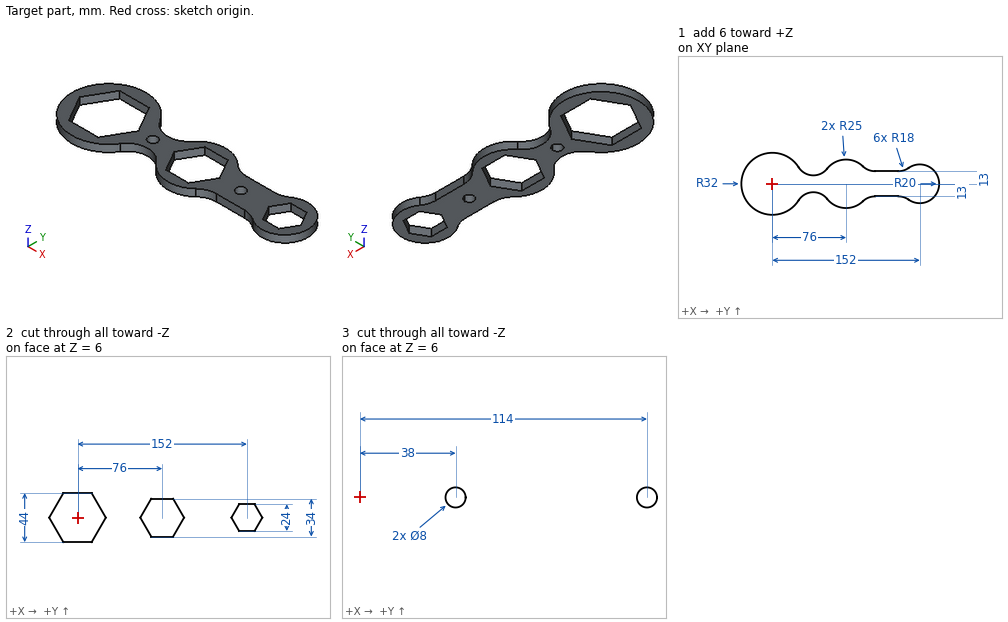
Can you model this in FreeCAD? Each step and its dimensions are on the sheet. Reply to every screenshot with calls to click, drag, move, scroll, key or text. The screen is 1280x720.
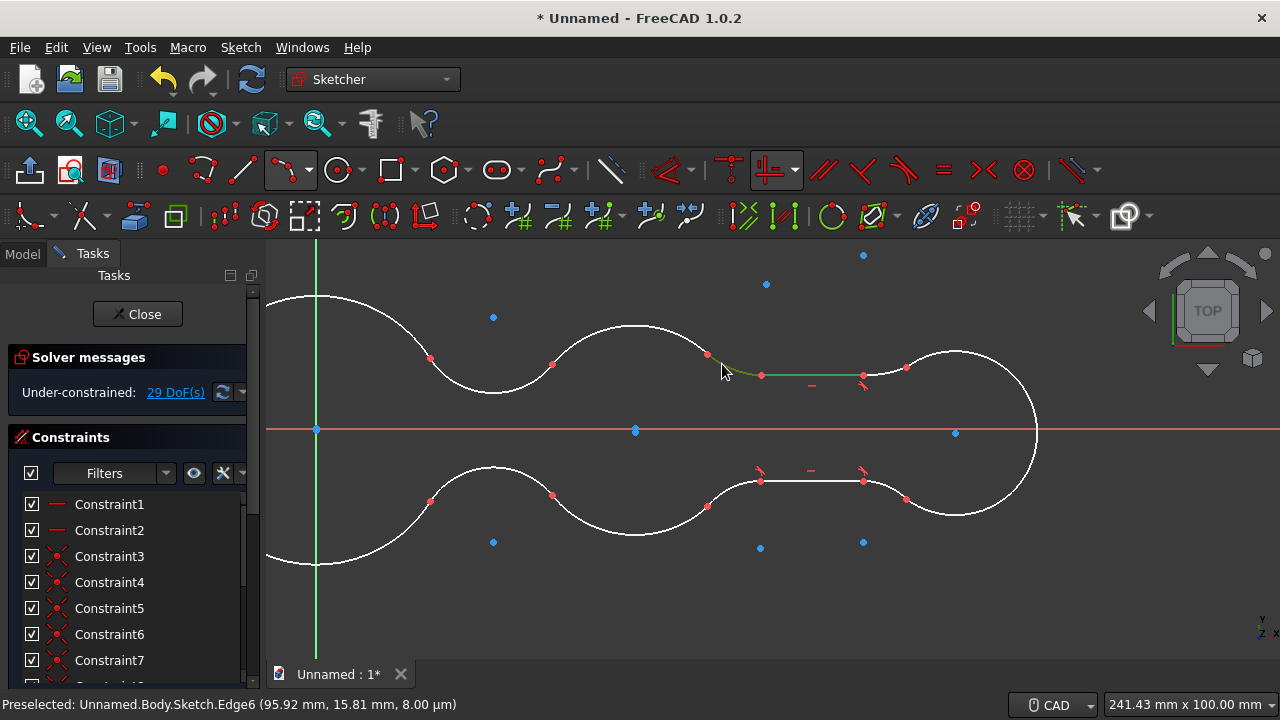
click(904, 170)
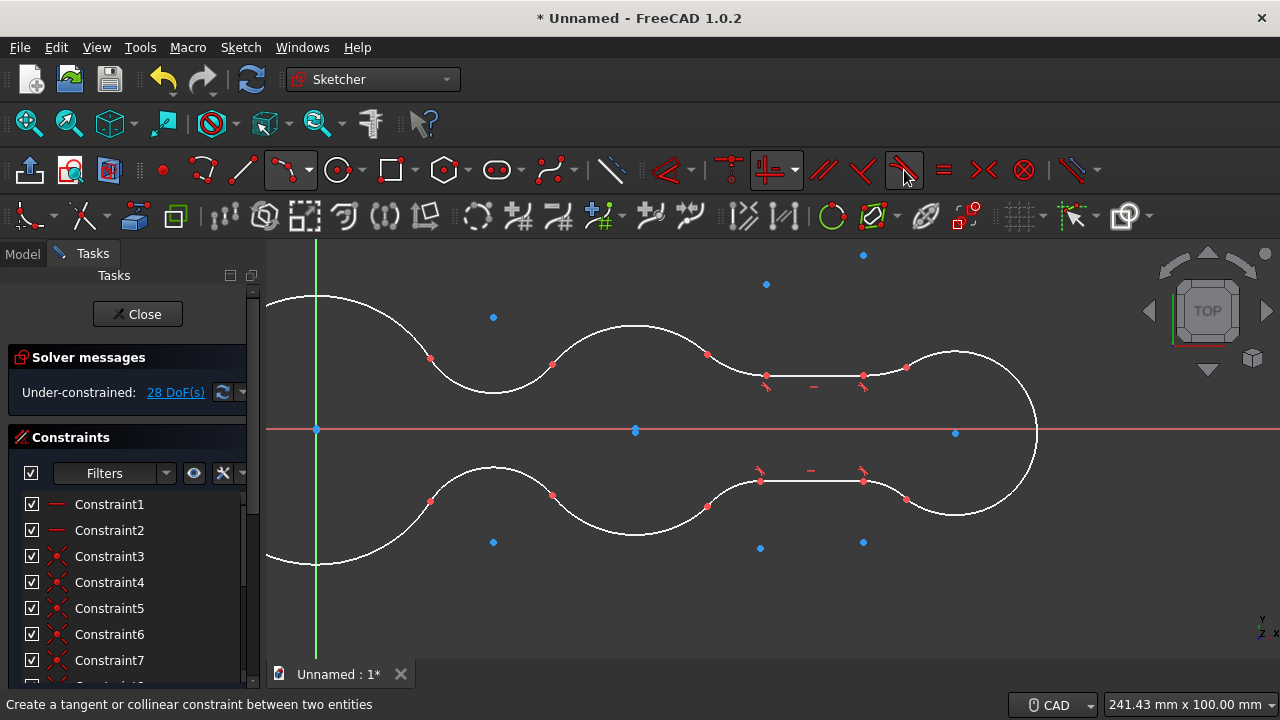
click(895, 490)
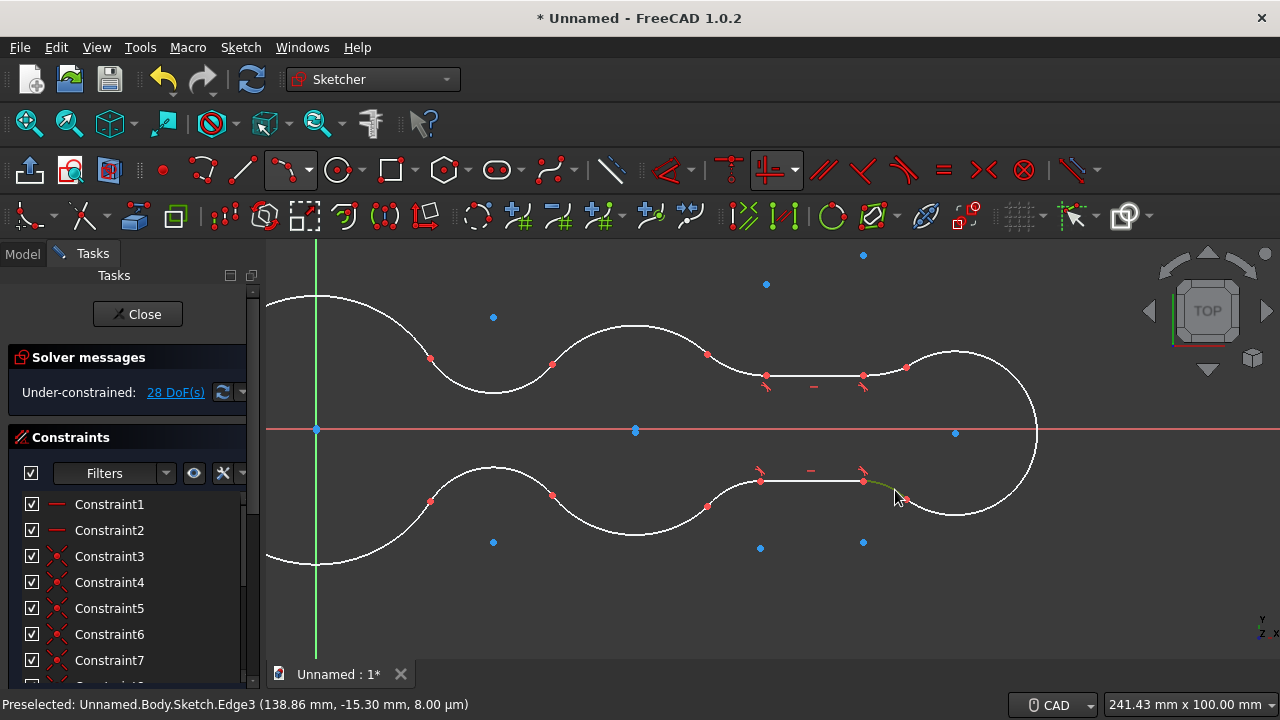
click(1007, 496)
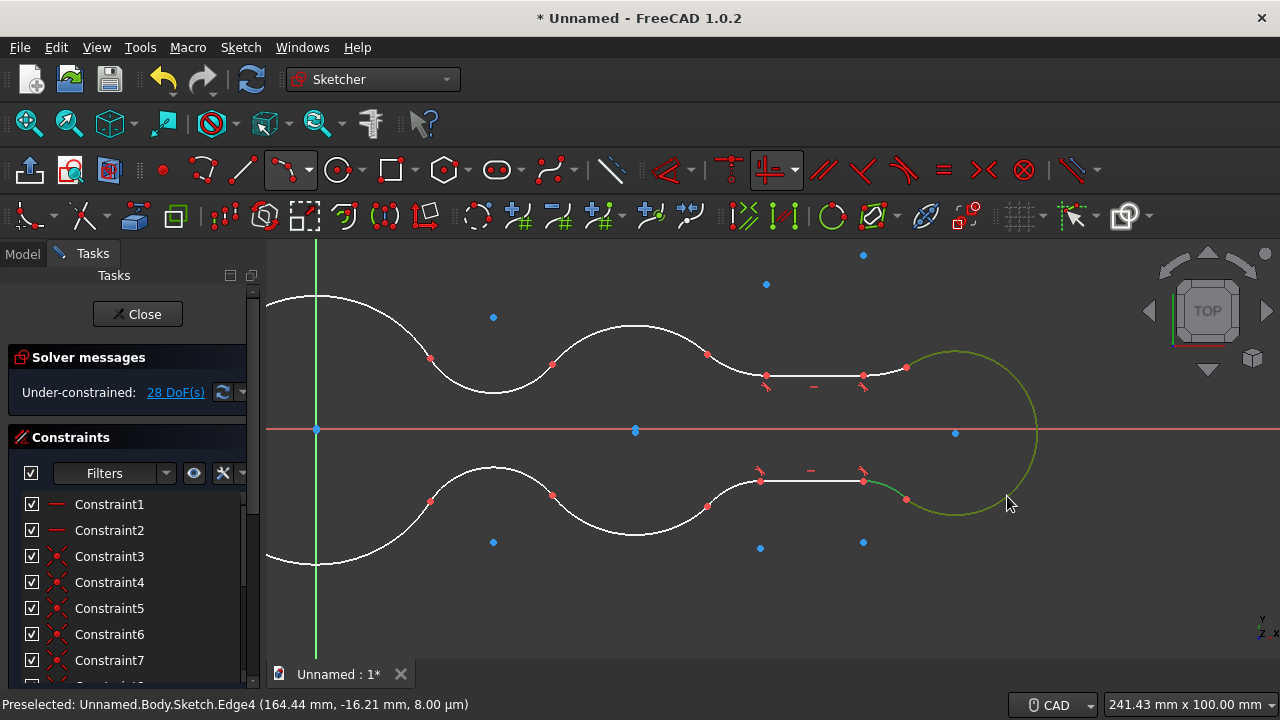
click(904, 170)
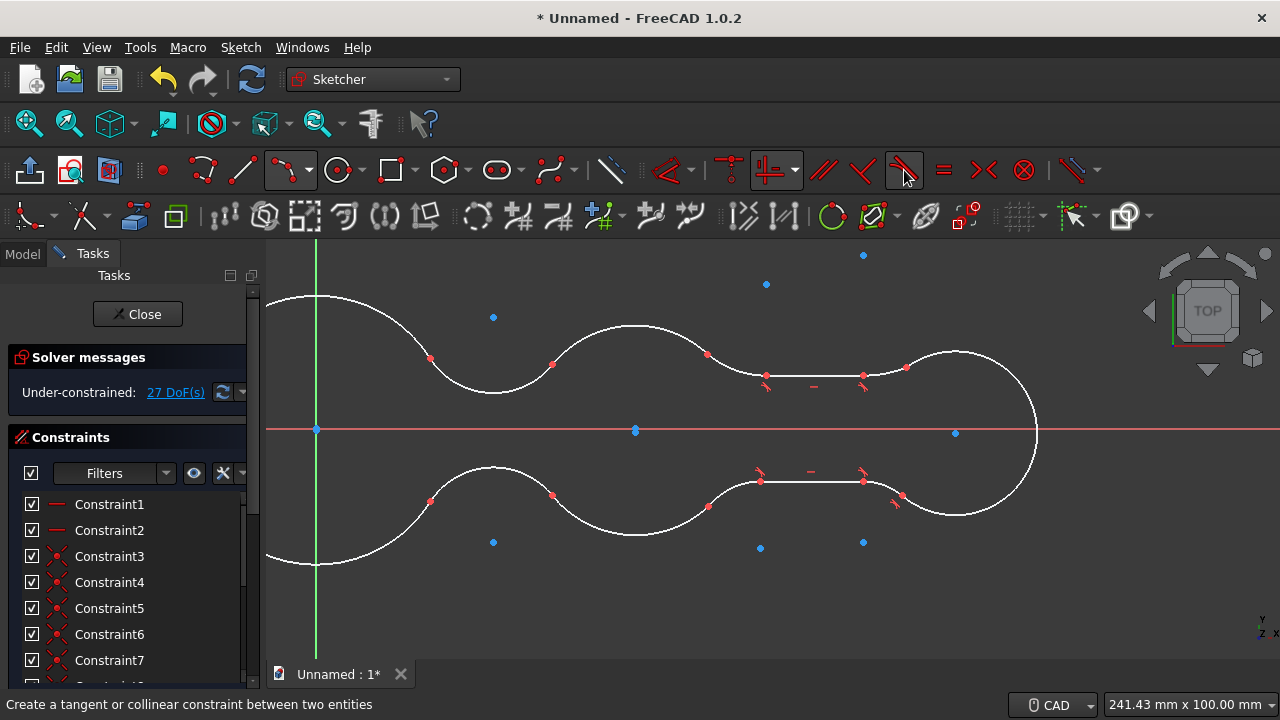
click(1004, 499)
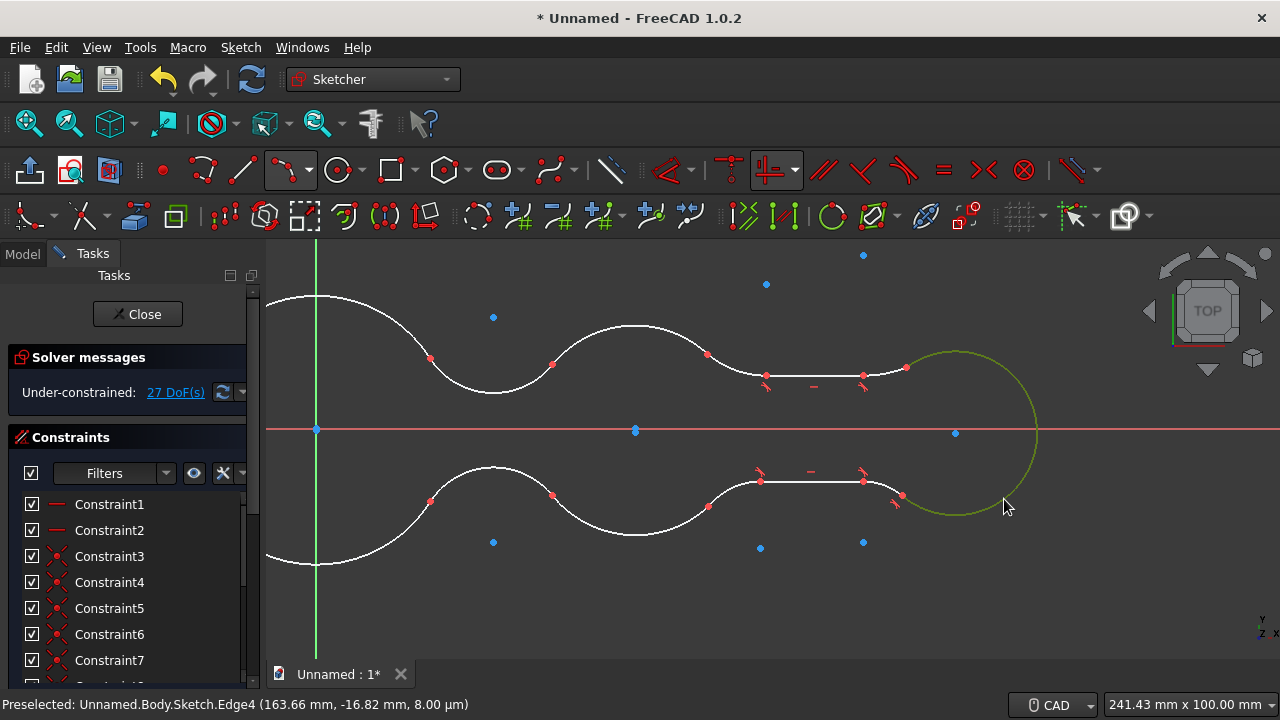
click(876, 375)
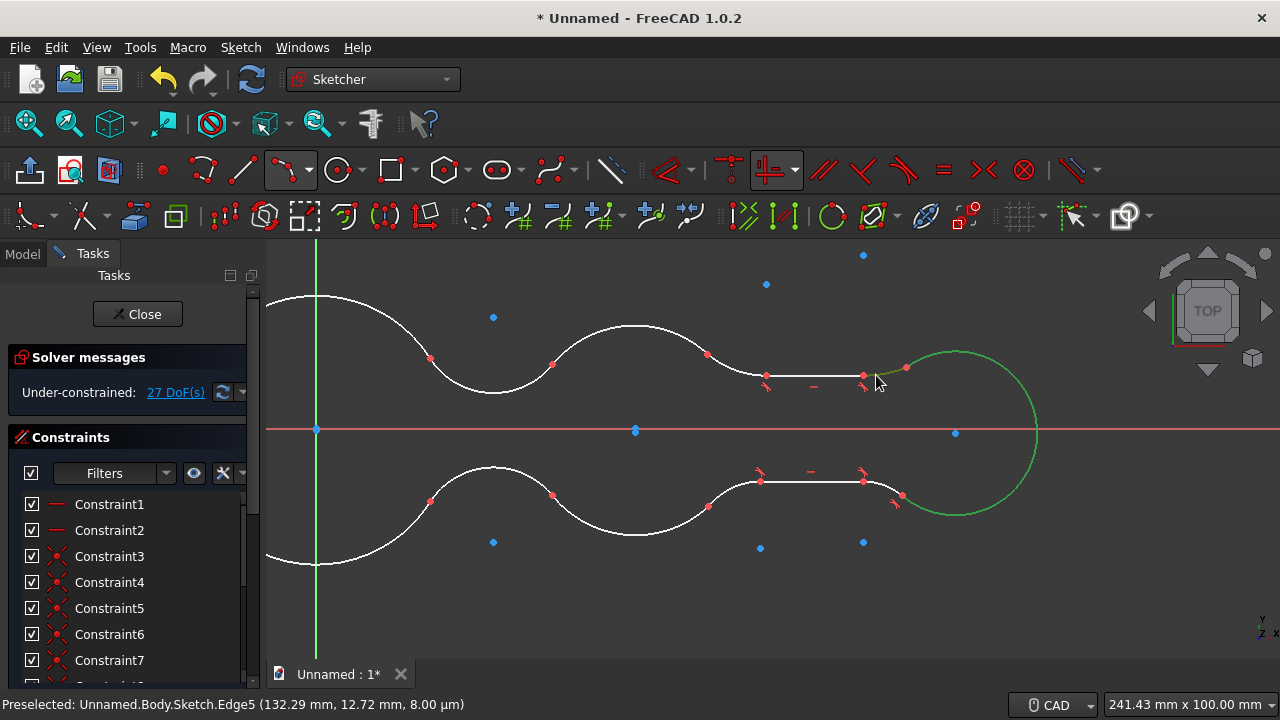
click(904, 170)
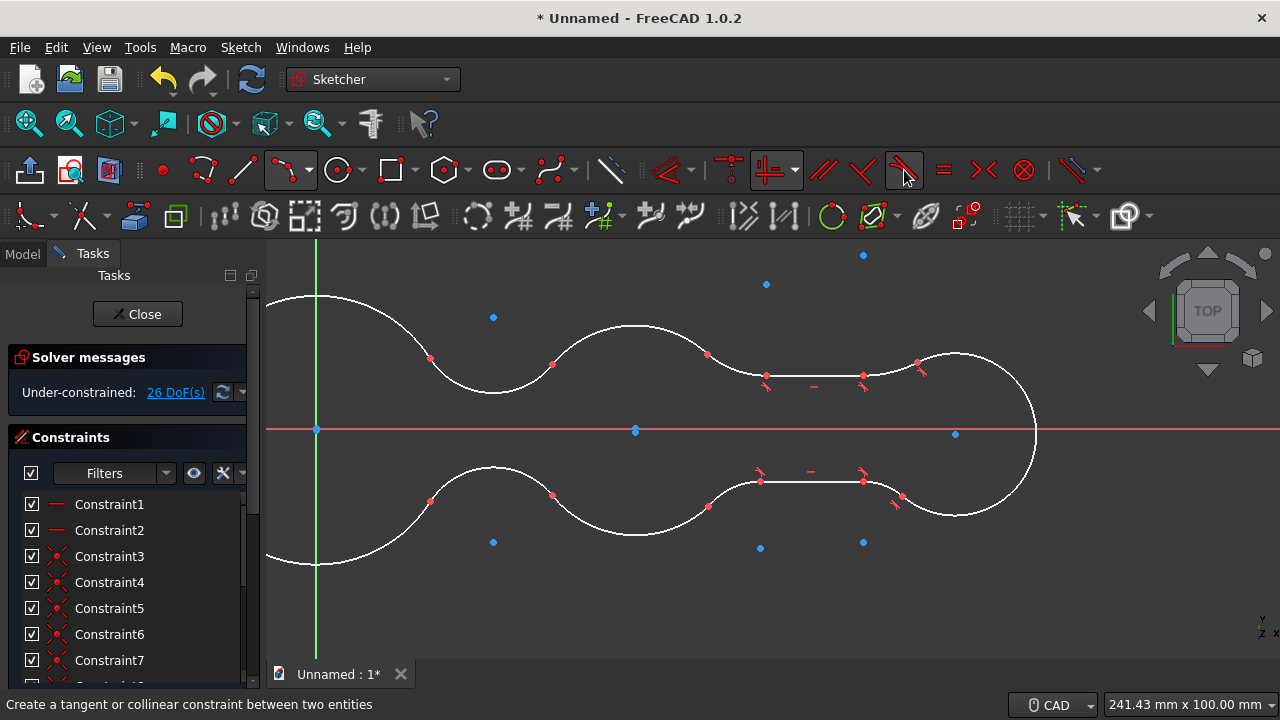
click(724, 365)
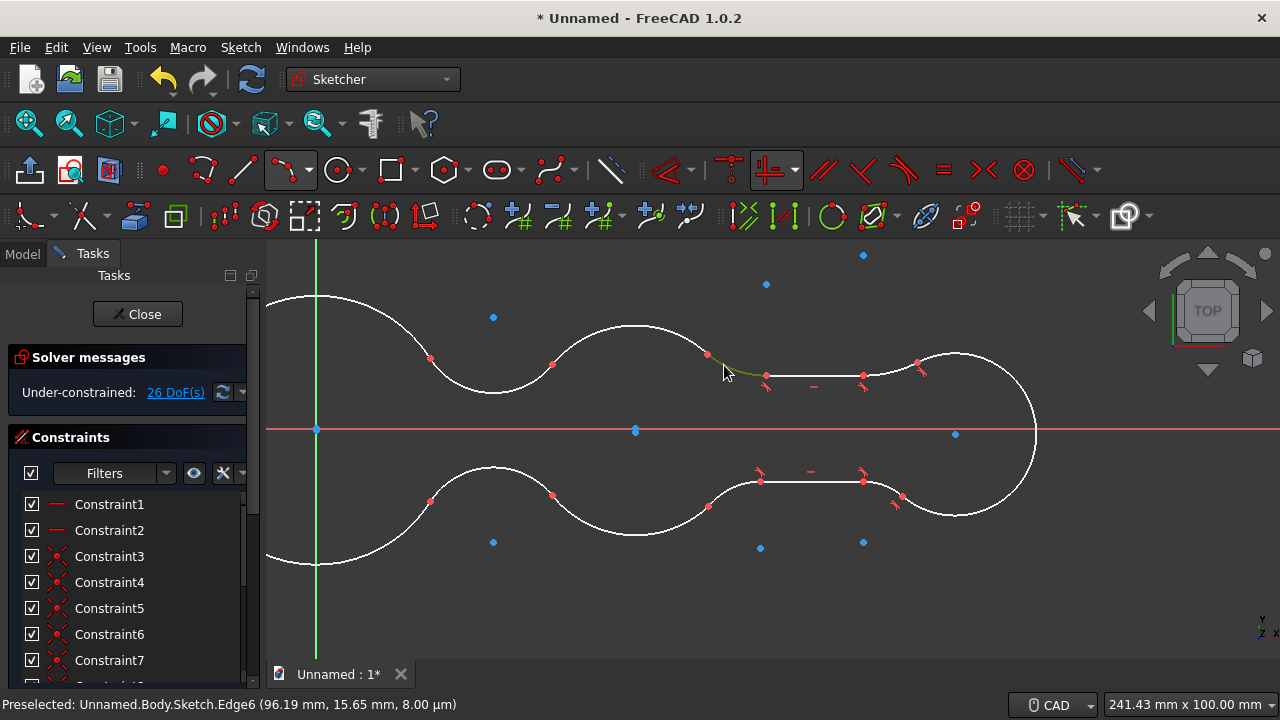
click(662, 329)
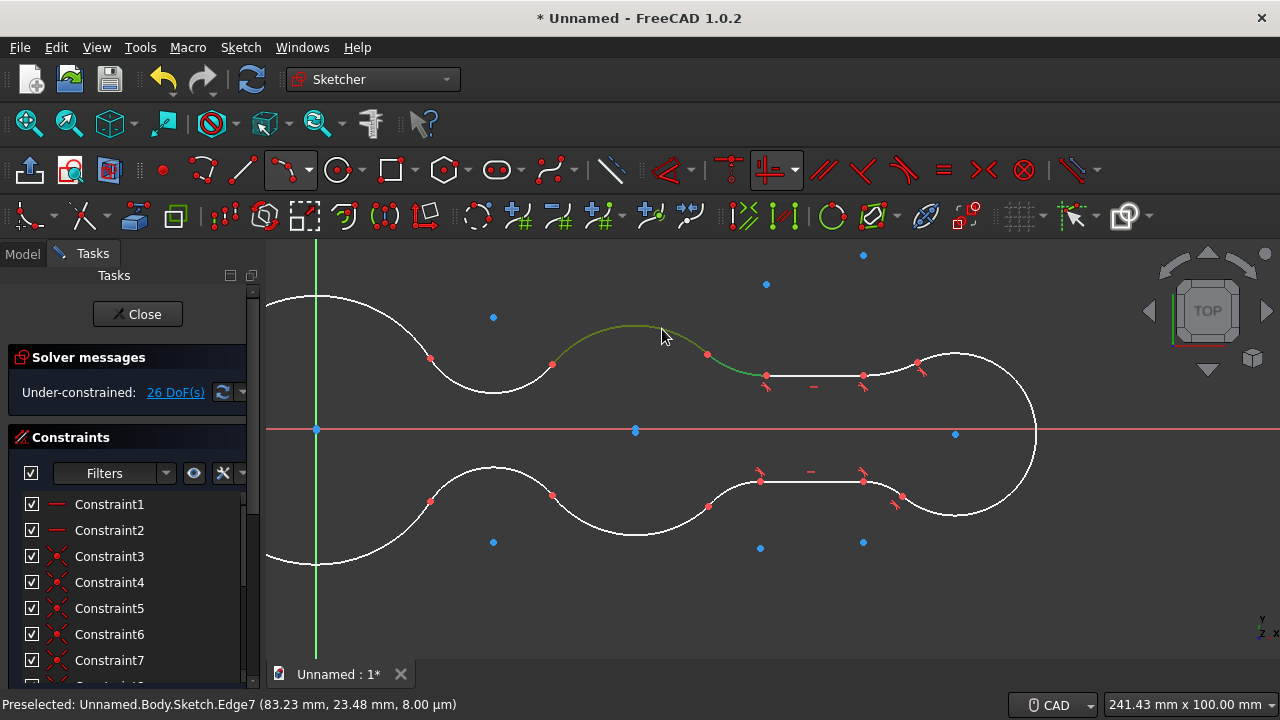
click(904, 170)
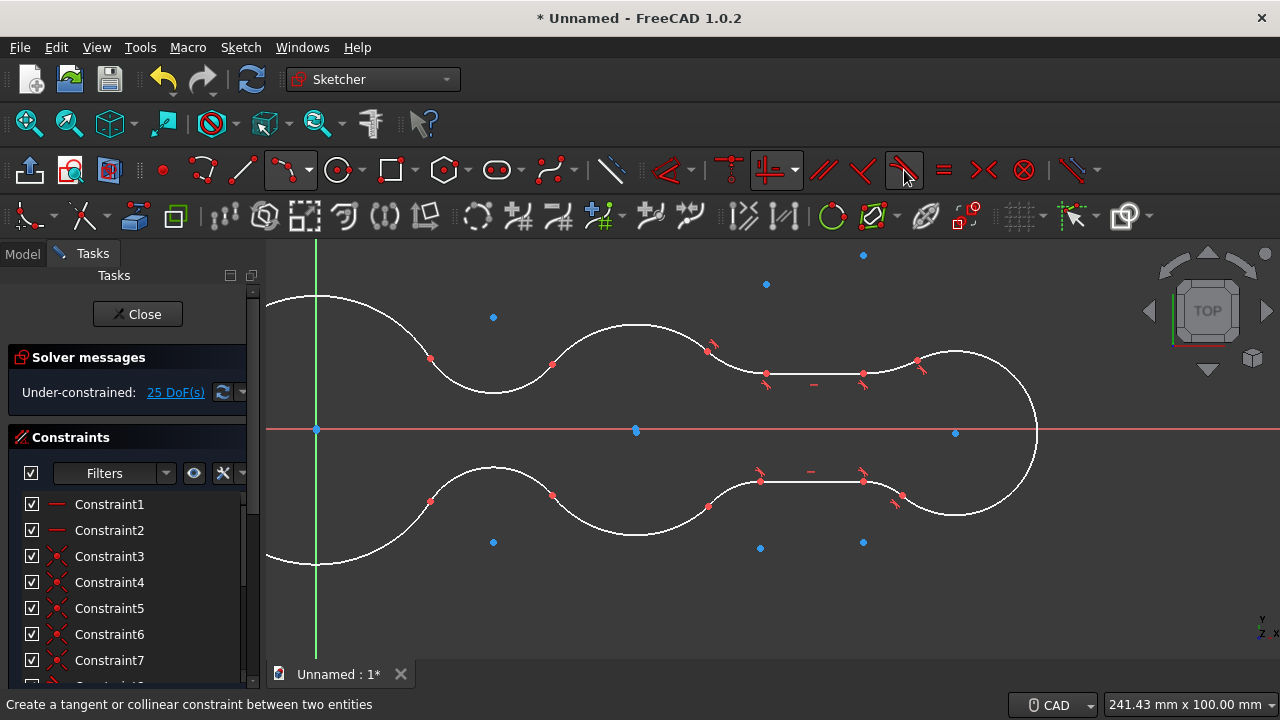
click(662, 328)